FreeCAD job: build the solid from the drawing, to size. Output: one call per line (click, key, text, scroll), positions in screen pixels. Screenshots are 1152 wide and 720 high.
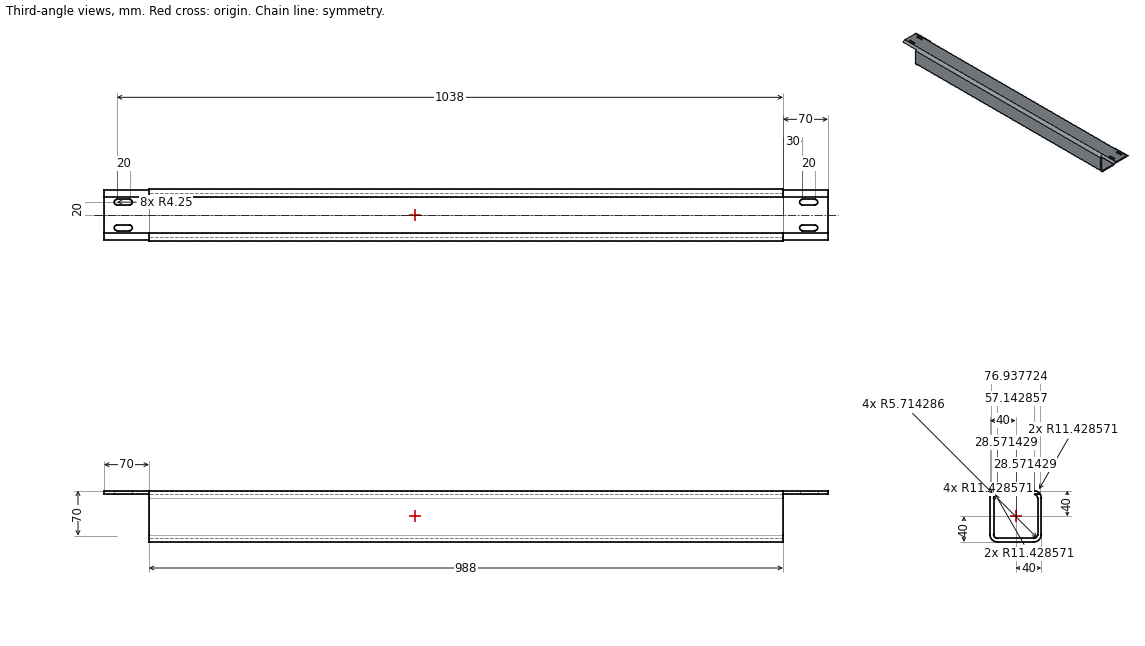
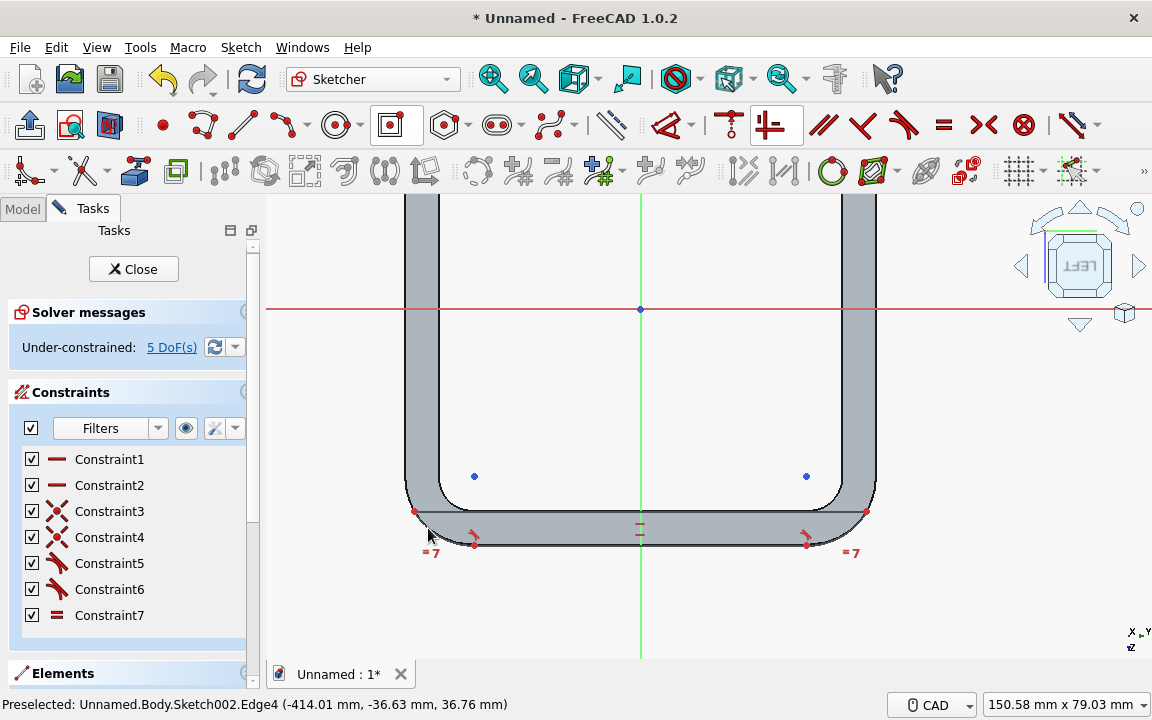
key(d)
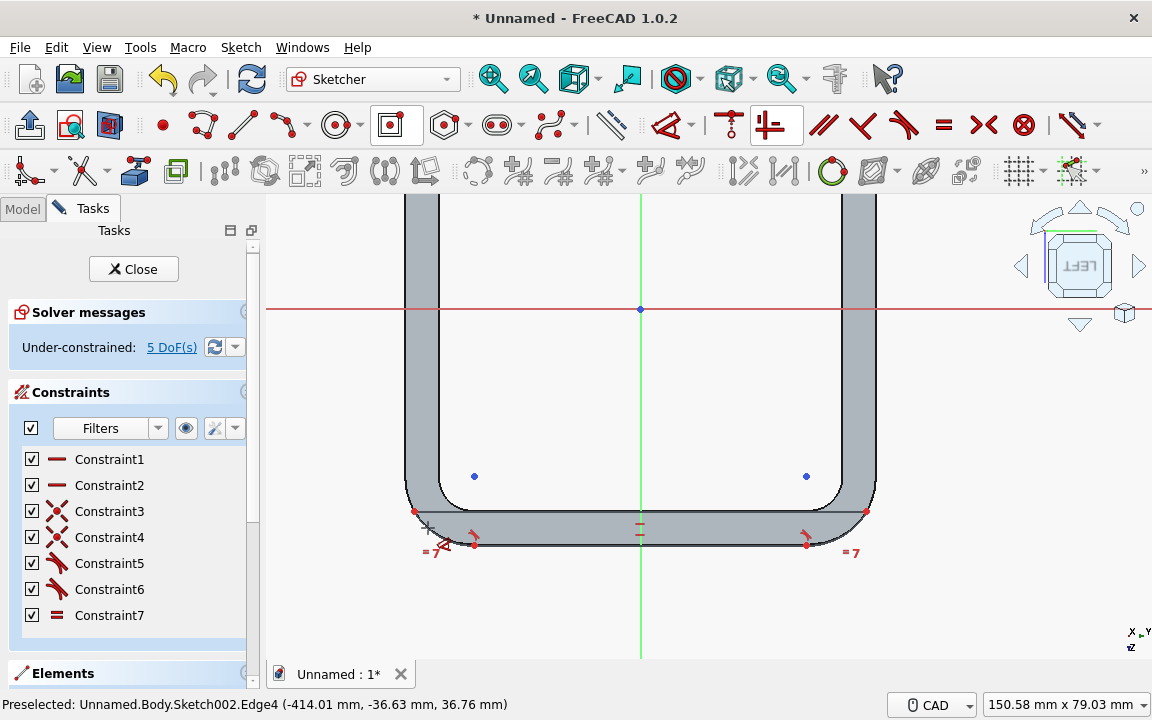
click(828, 543)
click(838, 574)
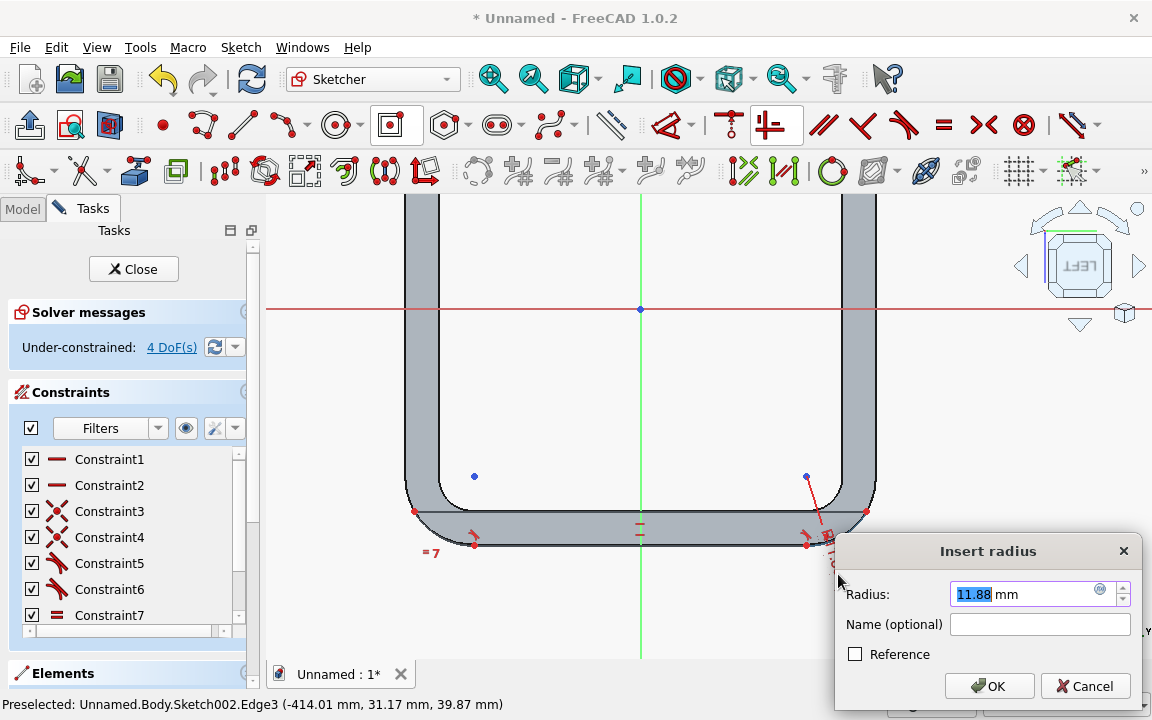
text(11.428571)
key(Return)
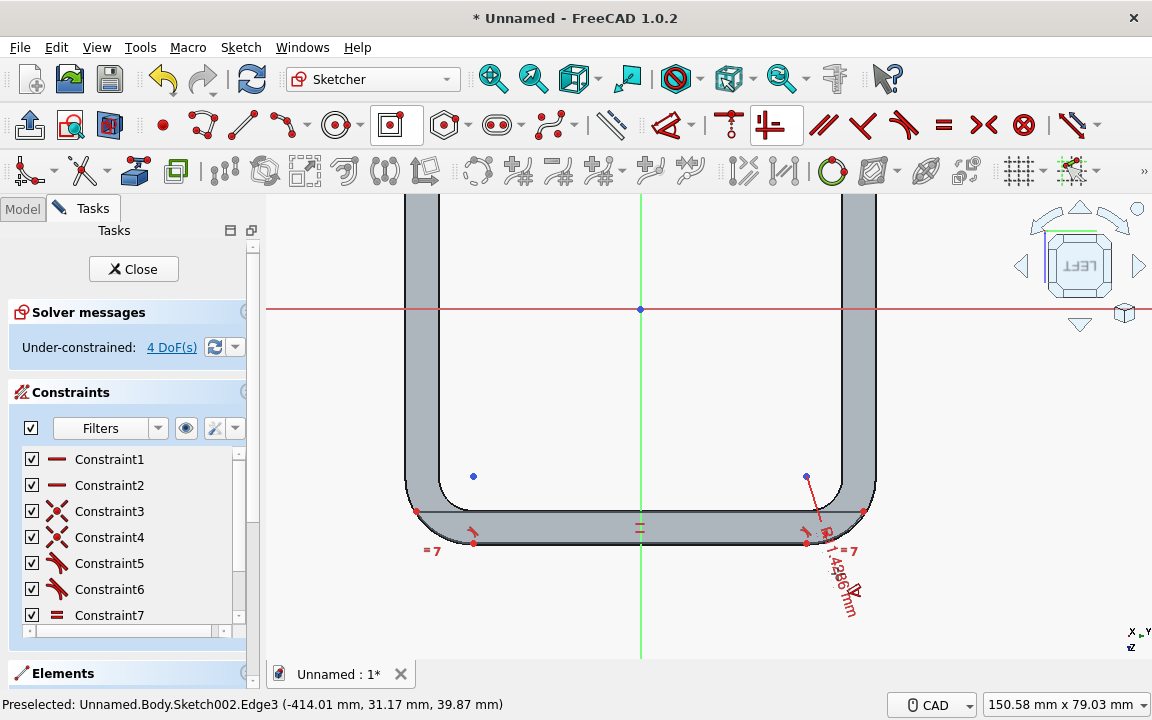
click(474, 543)
click(440, 426)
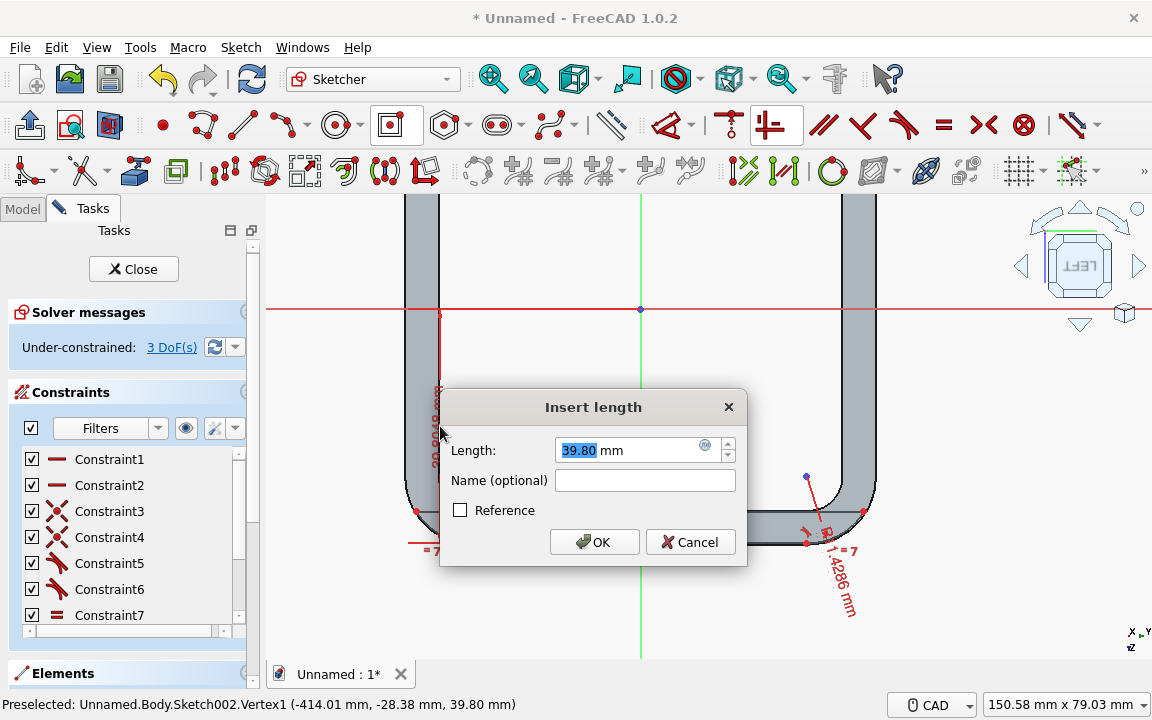
text(40)
key(Return)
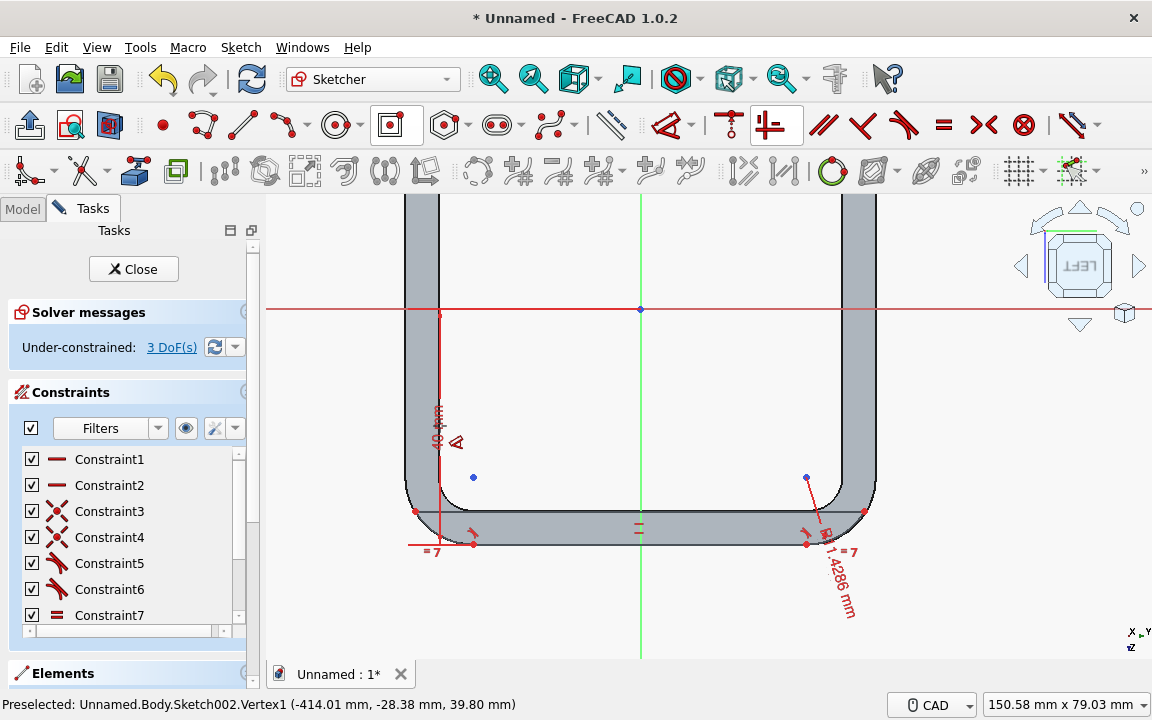
click(573, 545)
click(563, 579)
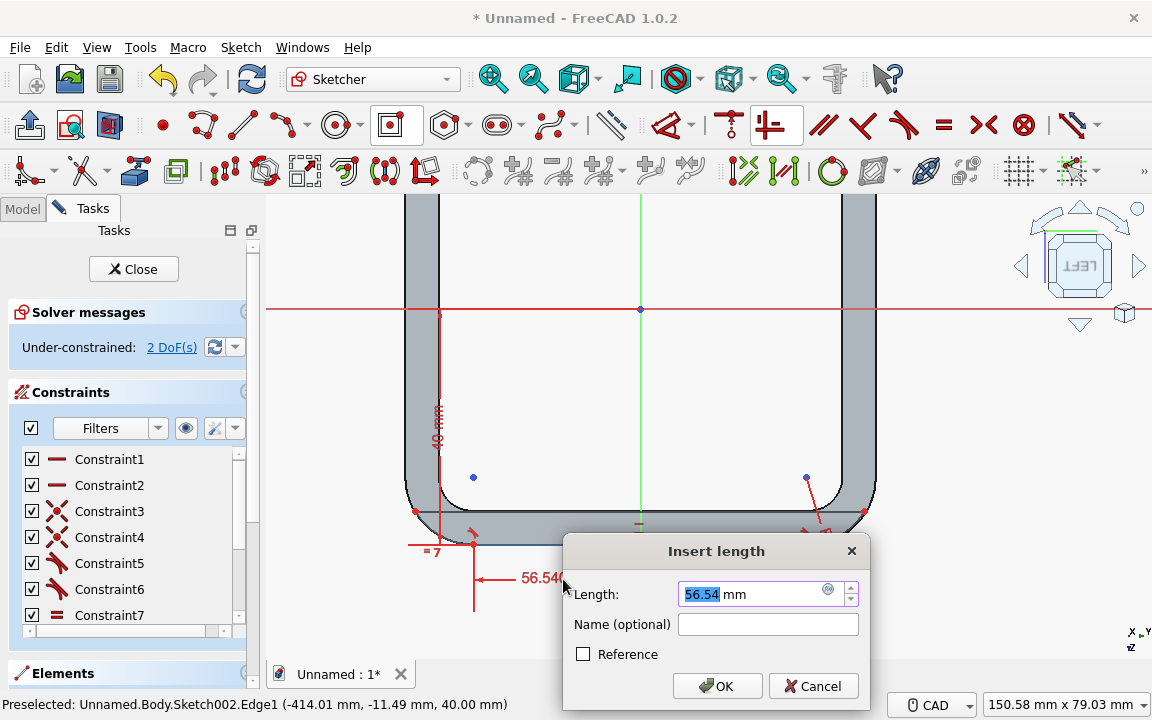
text(57.142857)
key(Return)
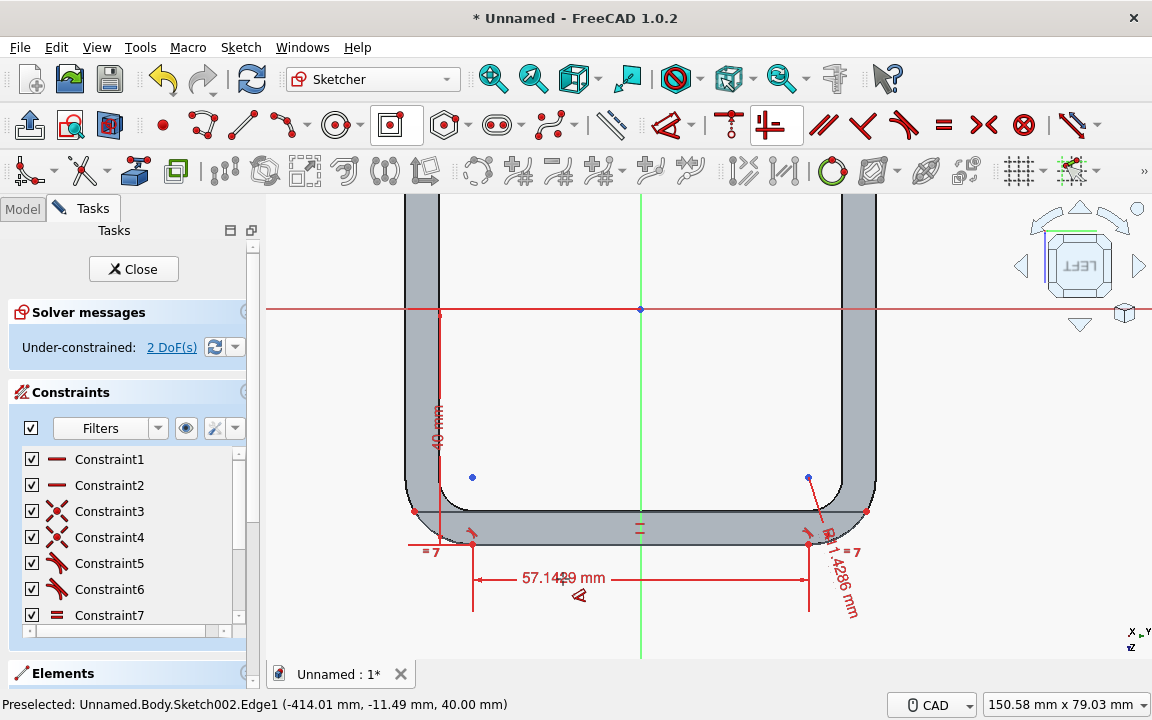
click(731, 512)
click(537, 478)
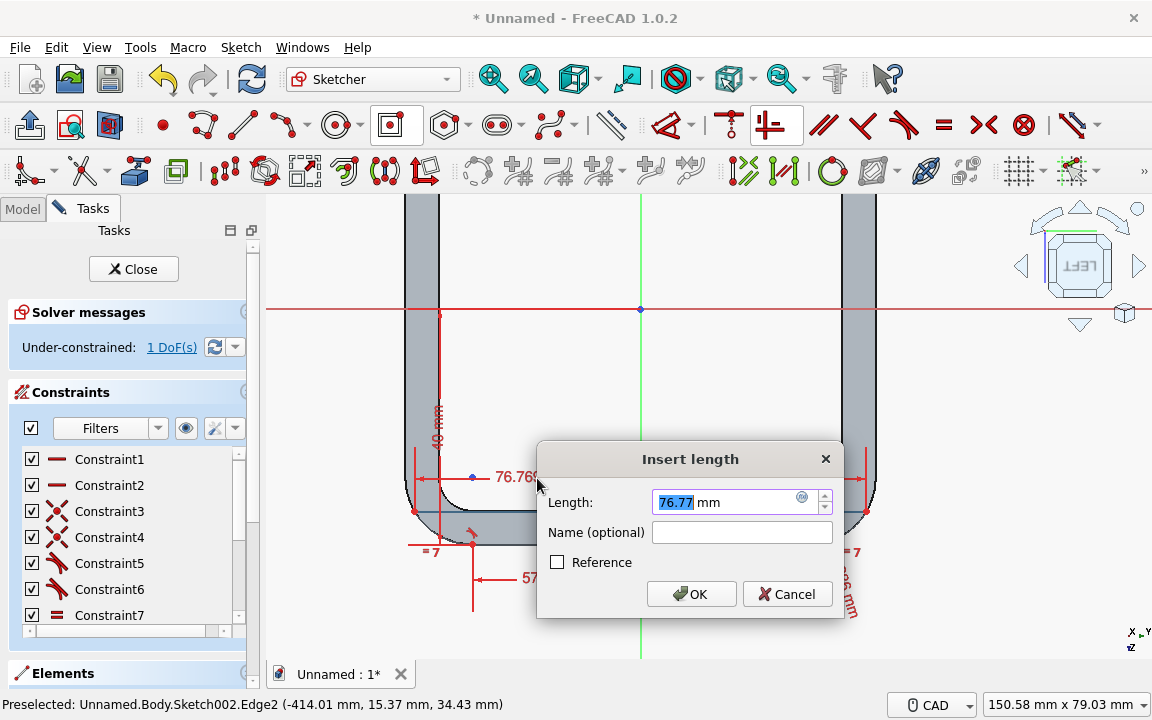
text(76.937724)
key(Return)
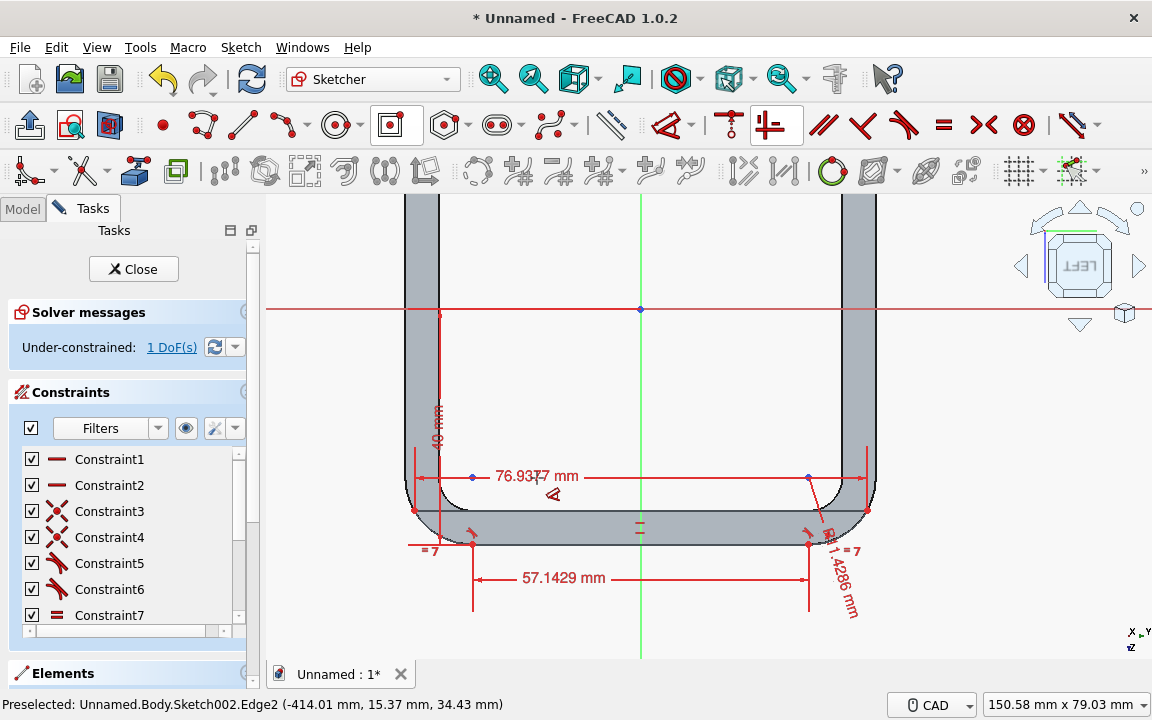
click(473, 545)
click(557, 275)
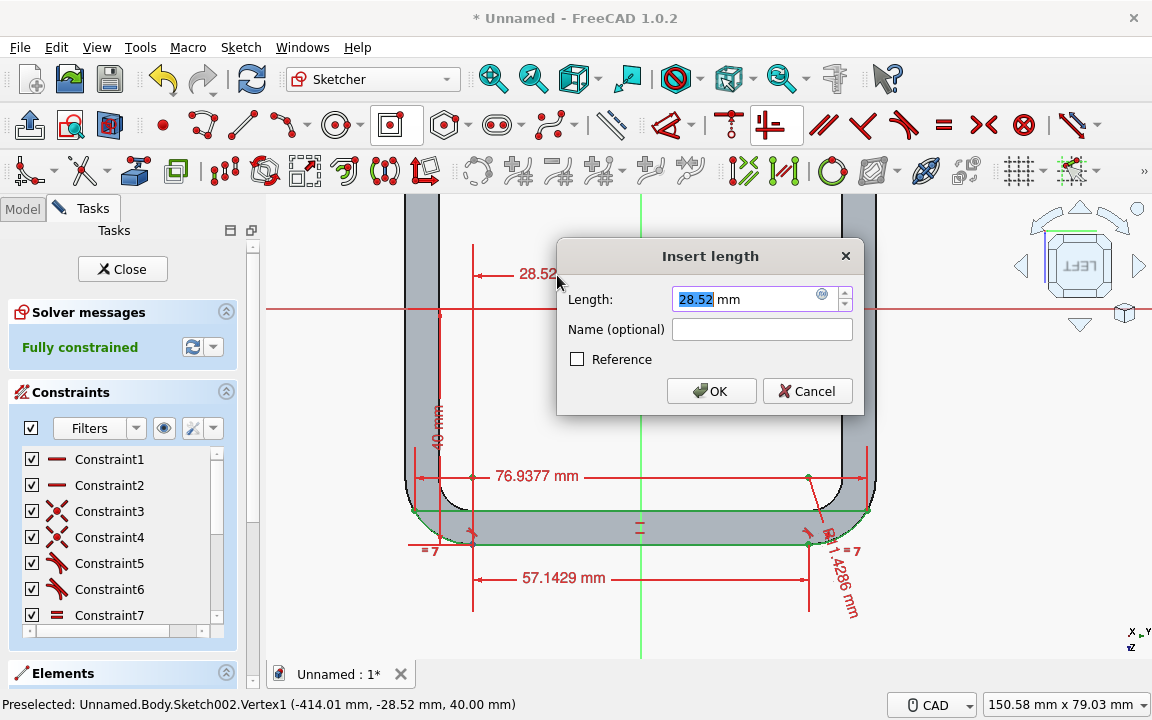
text(28.571429)
key(Return)
key(Escape)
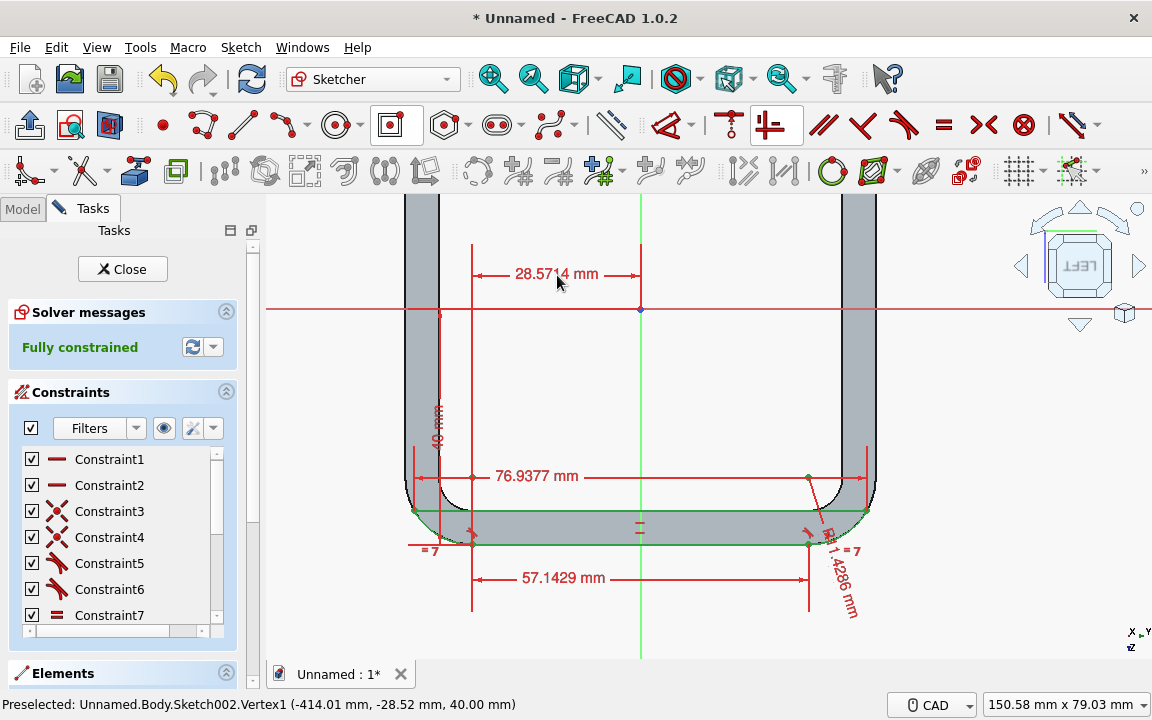
click(123, 269)